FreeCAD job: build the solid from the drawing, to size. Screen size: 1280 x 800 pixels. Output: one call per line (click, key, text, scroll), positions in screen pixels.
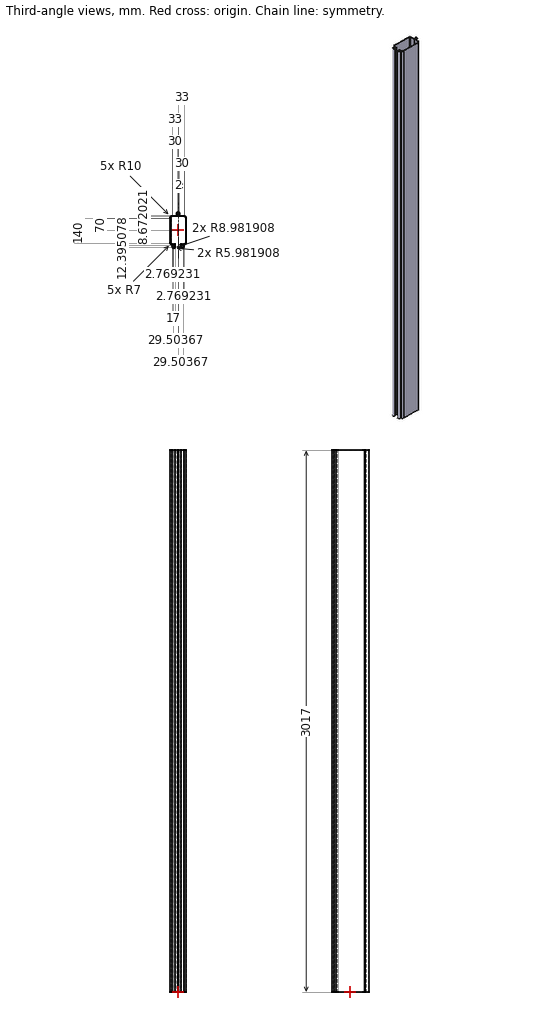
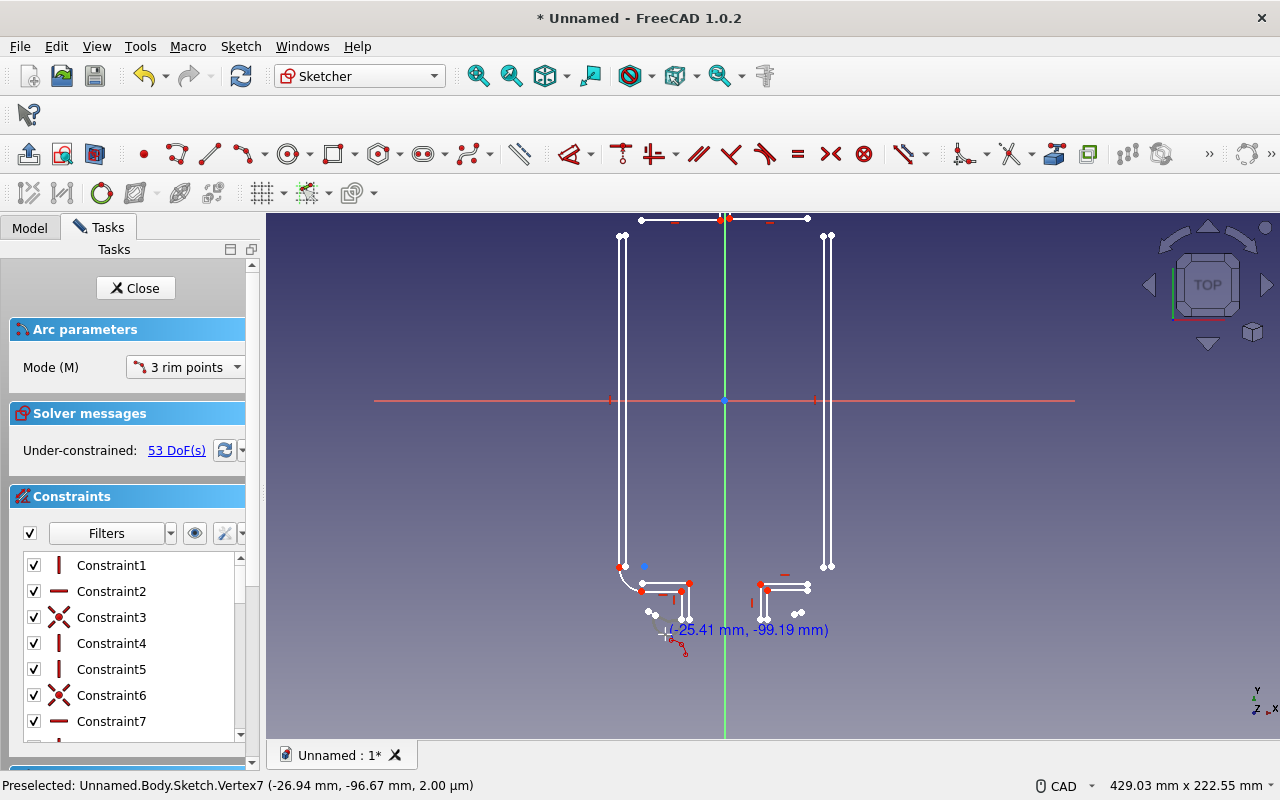
click(665, 633)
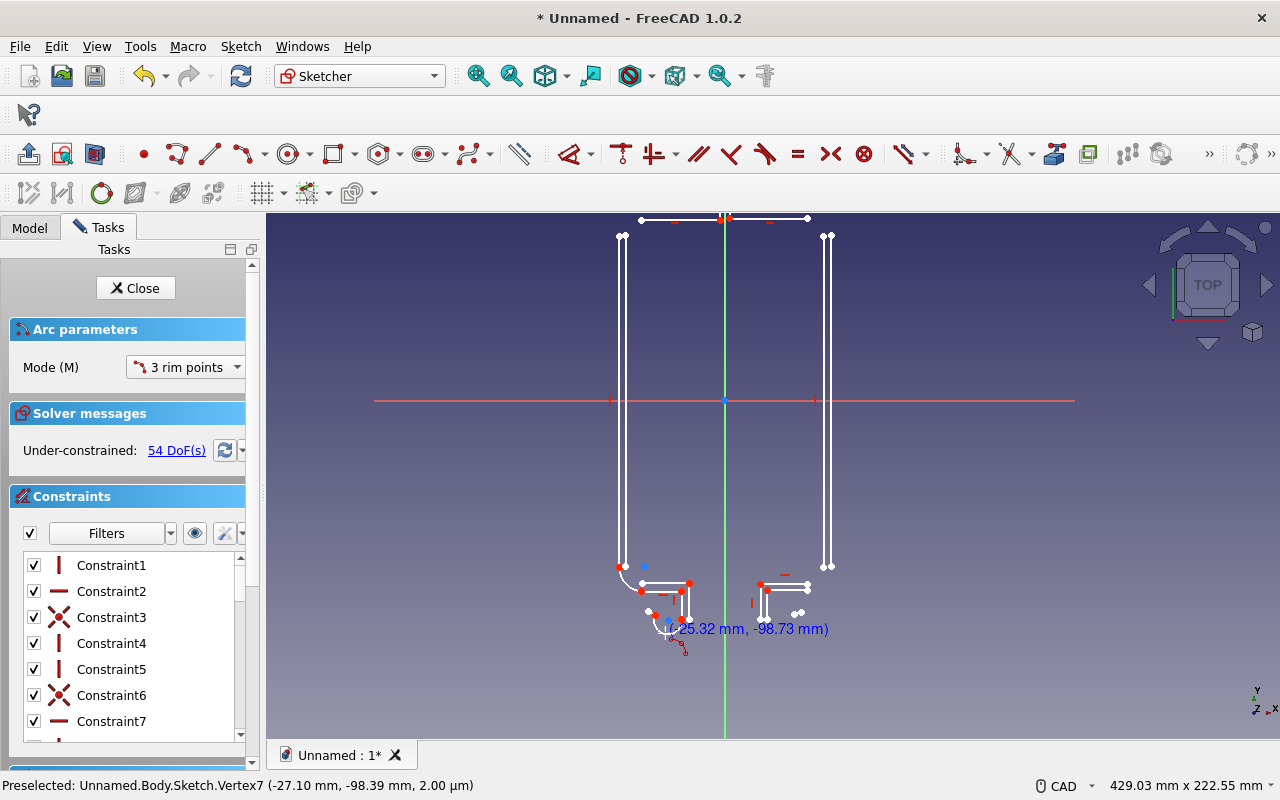
scroll(649, 611, up, 8)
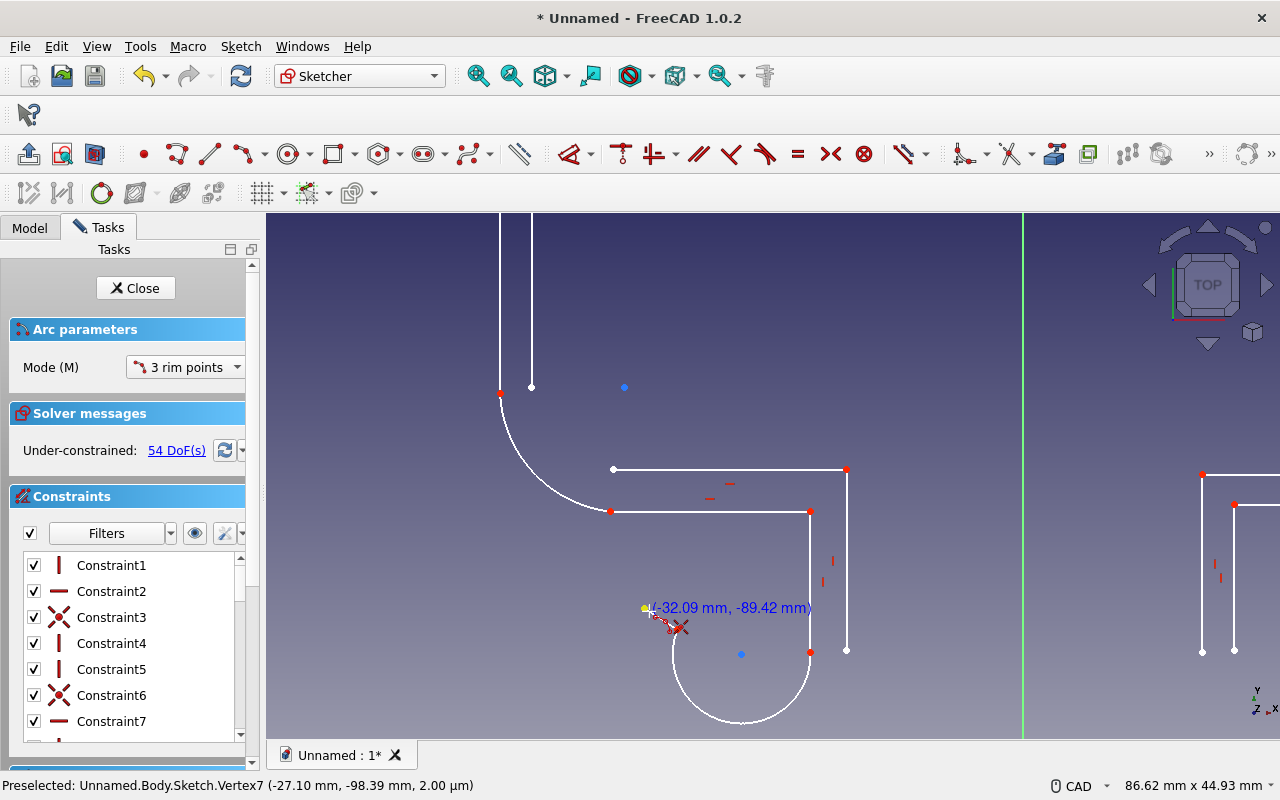
click(645, 608)
click(847, 650)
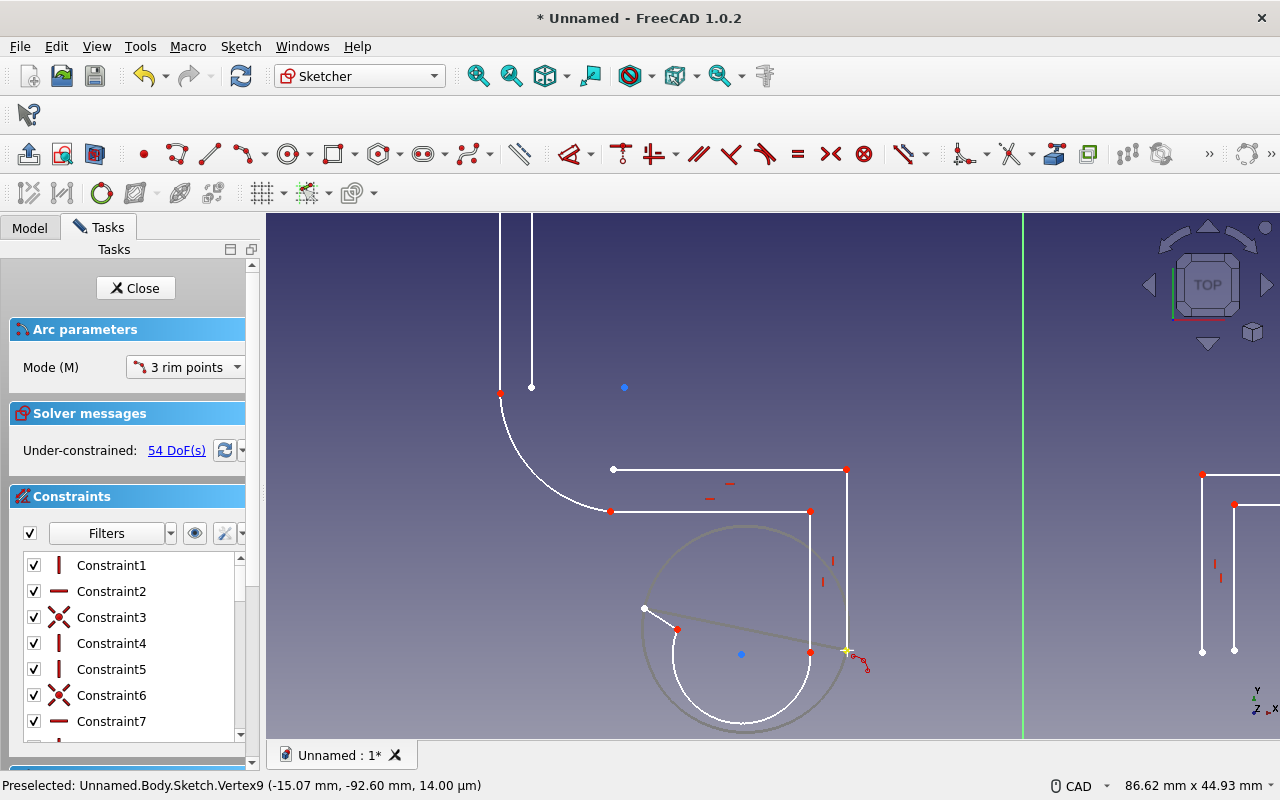
scroll(655, 619, down, 10)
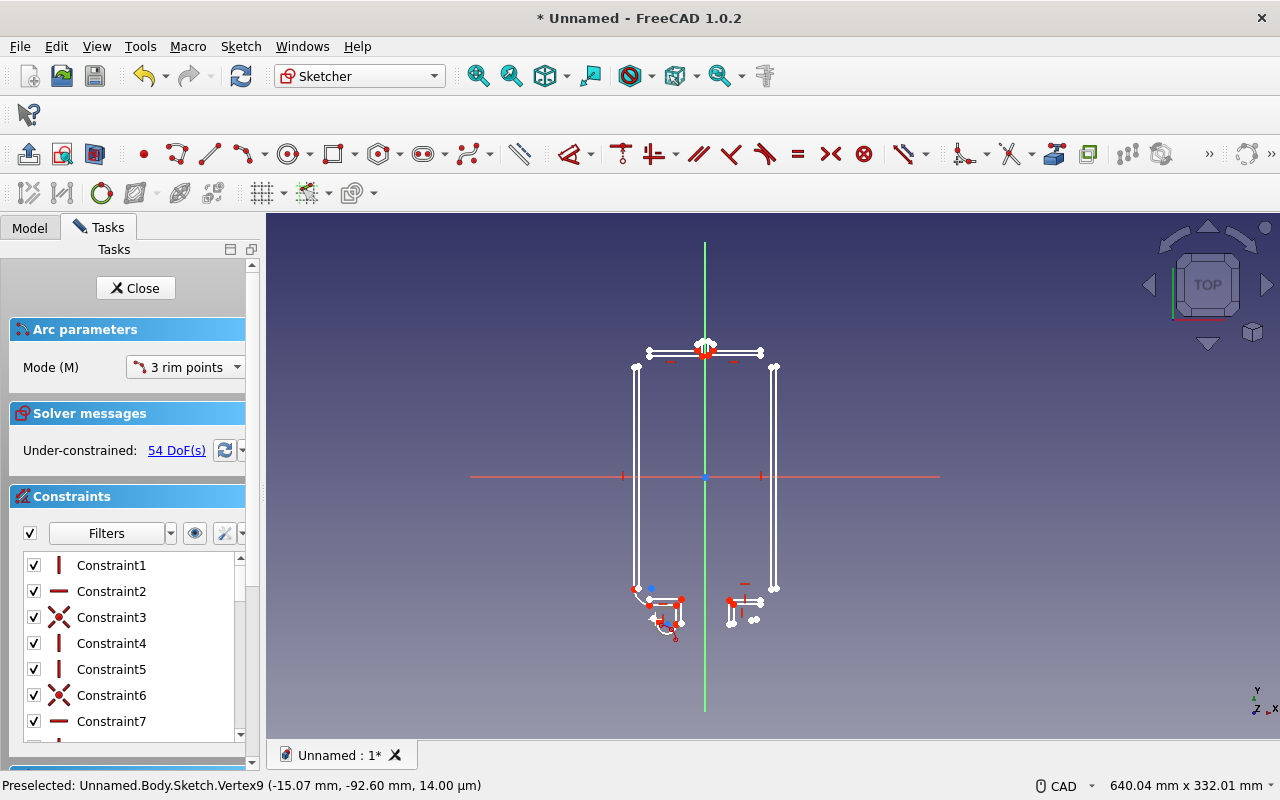
scroll(674, 636, up, 7)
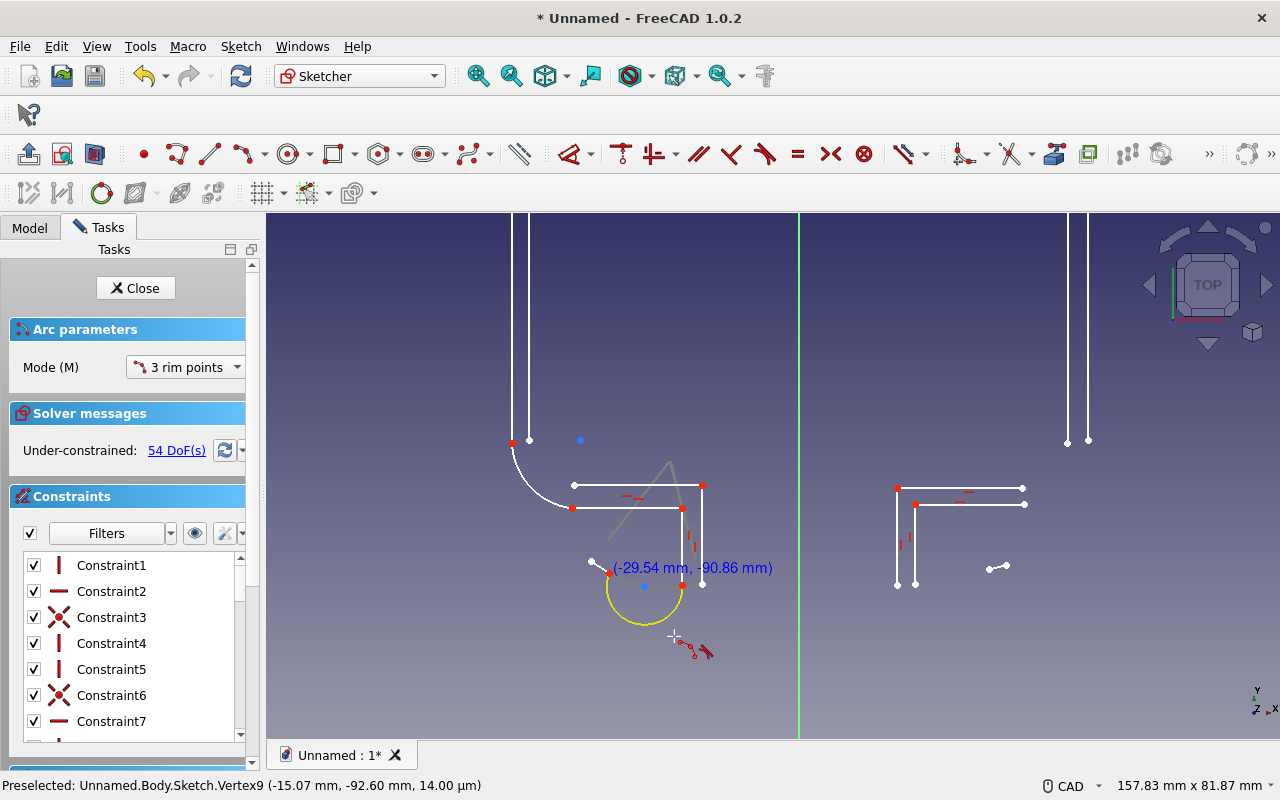
click(673, 633)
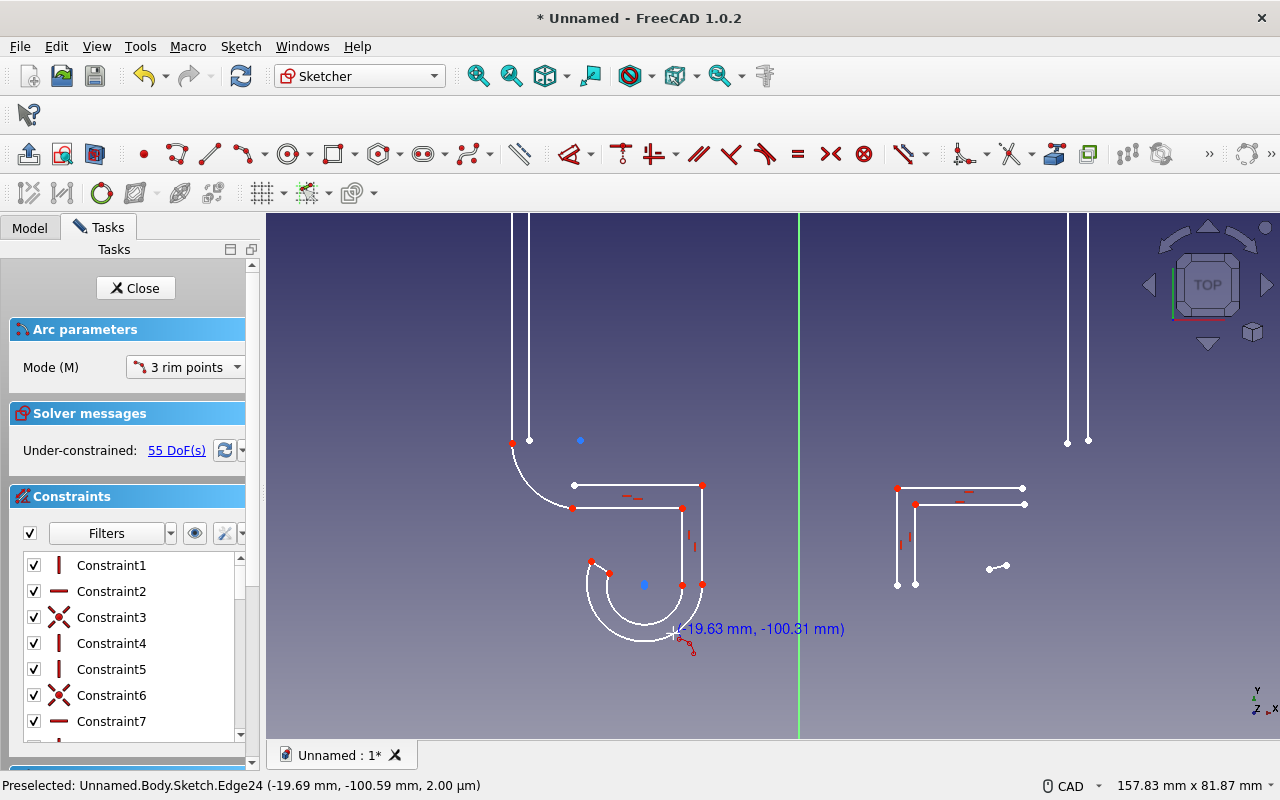
click(574, 485)
click(529, 440)
click(542, 471)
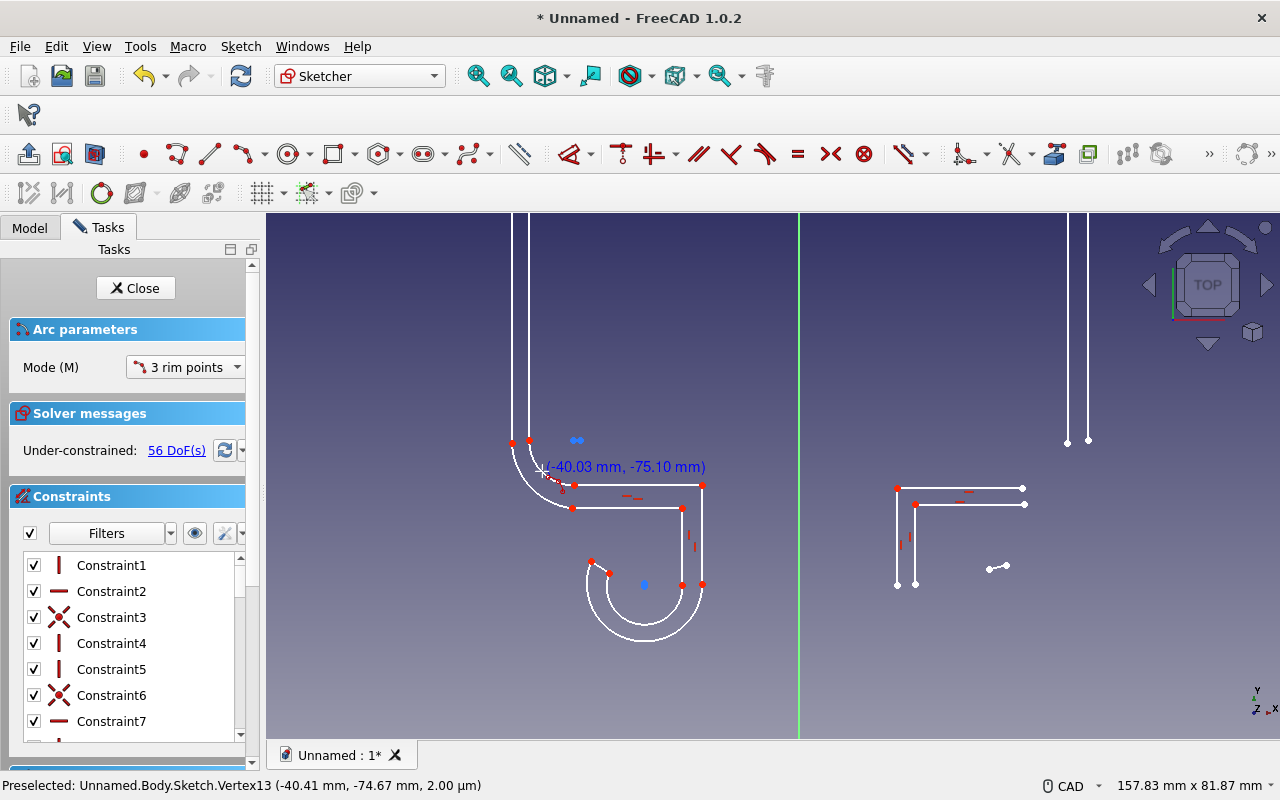
scroll(674, 636, down, 7)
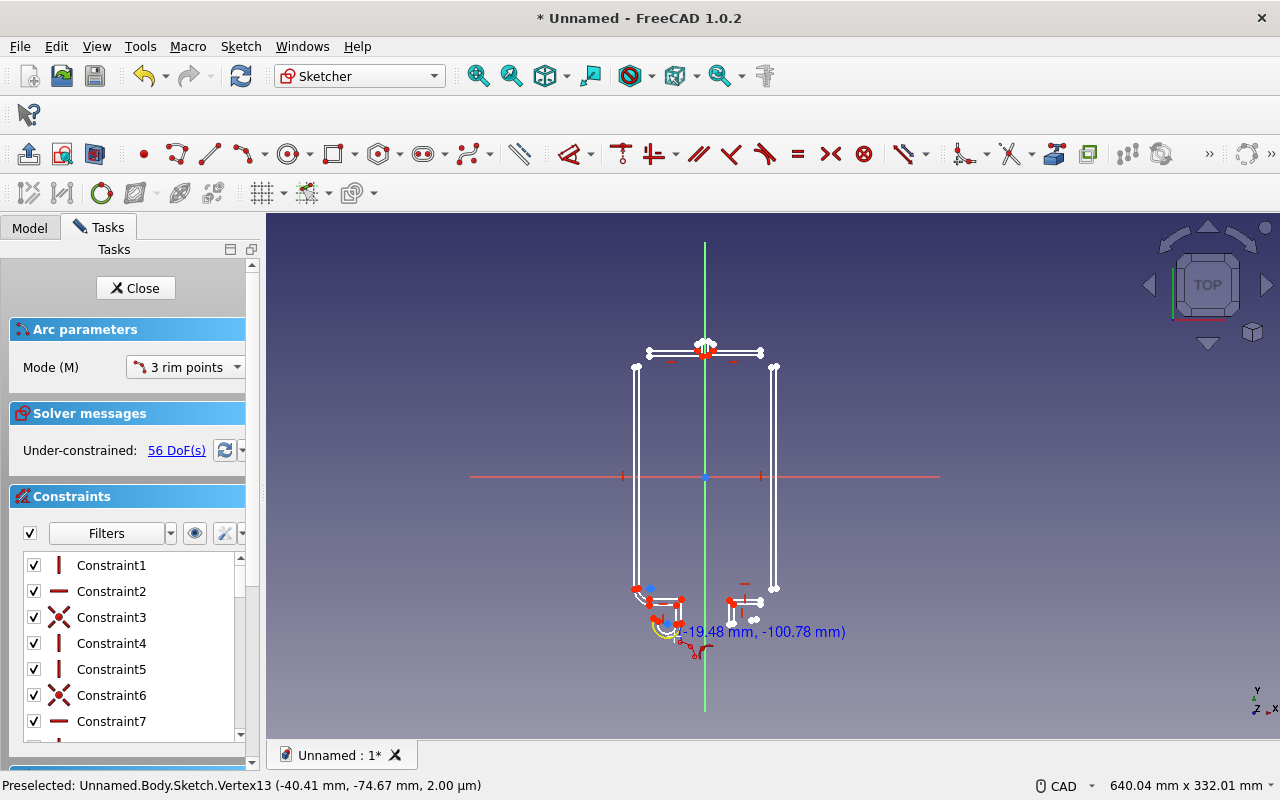
scroll(639, 366, up, 7)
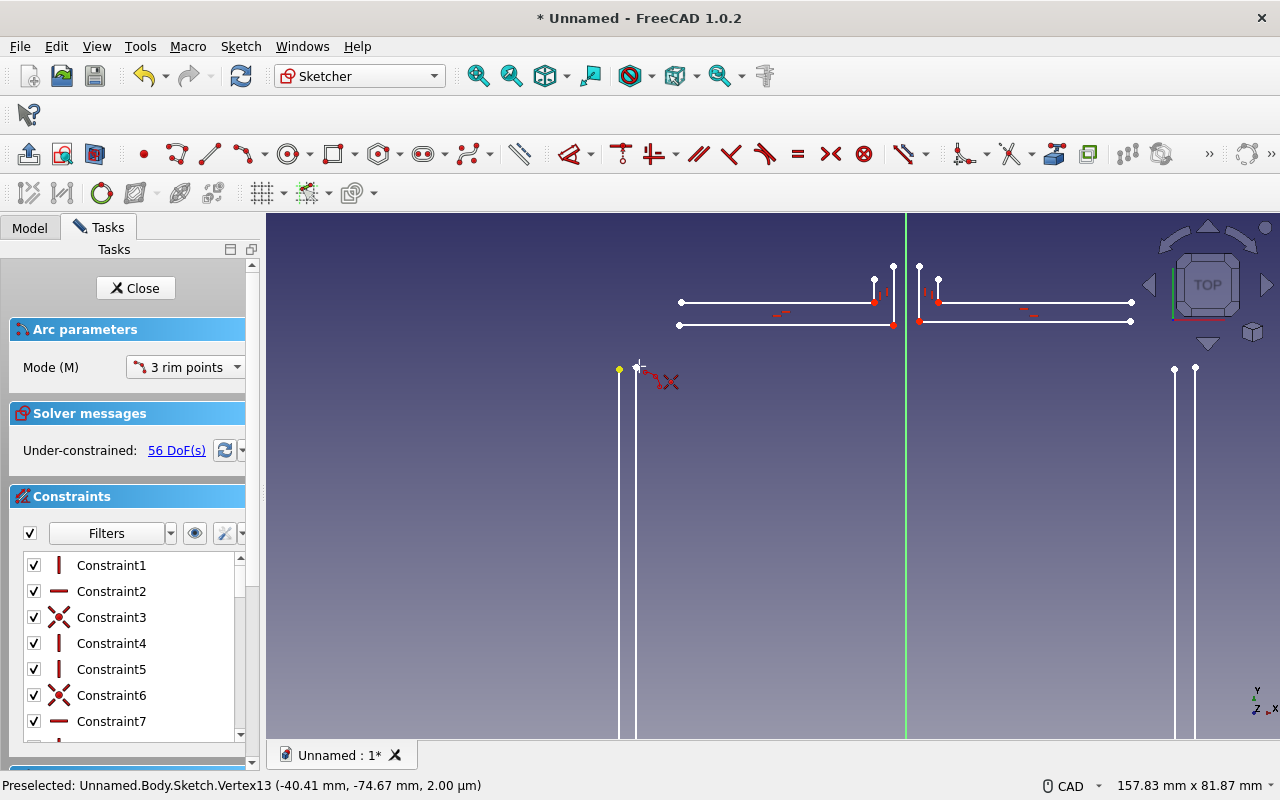
click(636, 368)
click(680, 325)
click(650, 334)